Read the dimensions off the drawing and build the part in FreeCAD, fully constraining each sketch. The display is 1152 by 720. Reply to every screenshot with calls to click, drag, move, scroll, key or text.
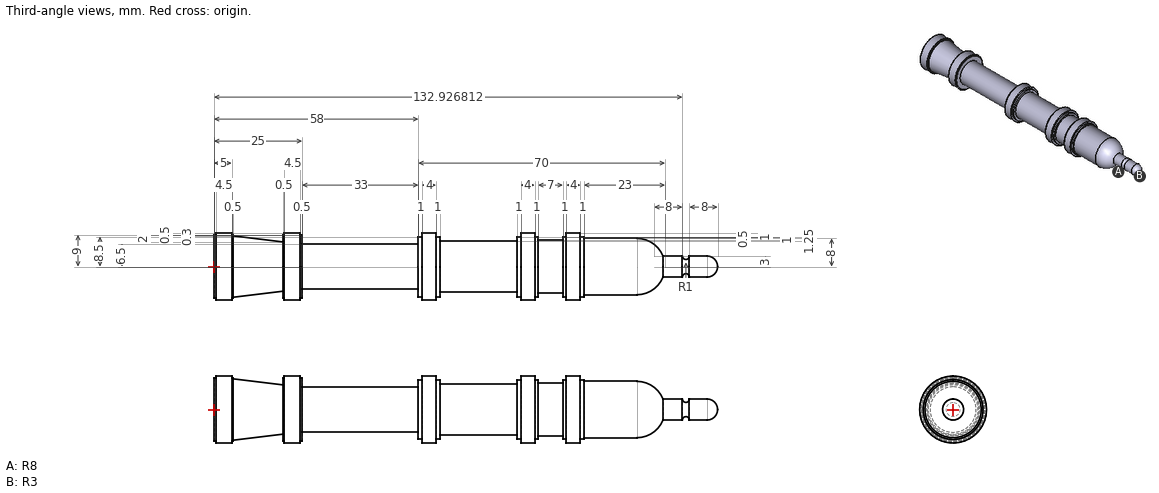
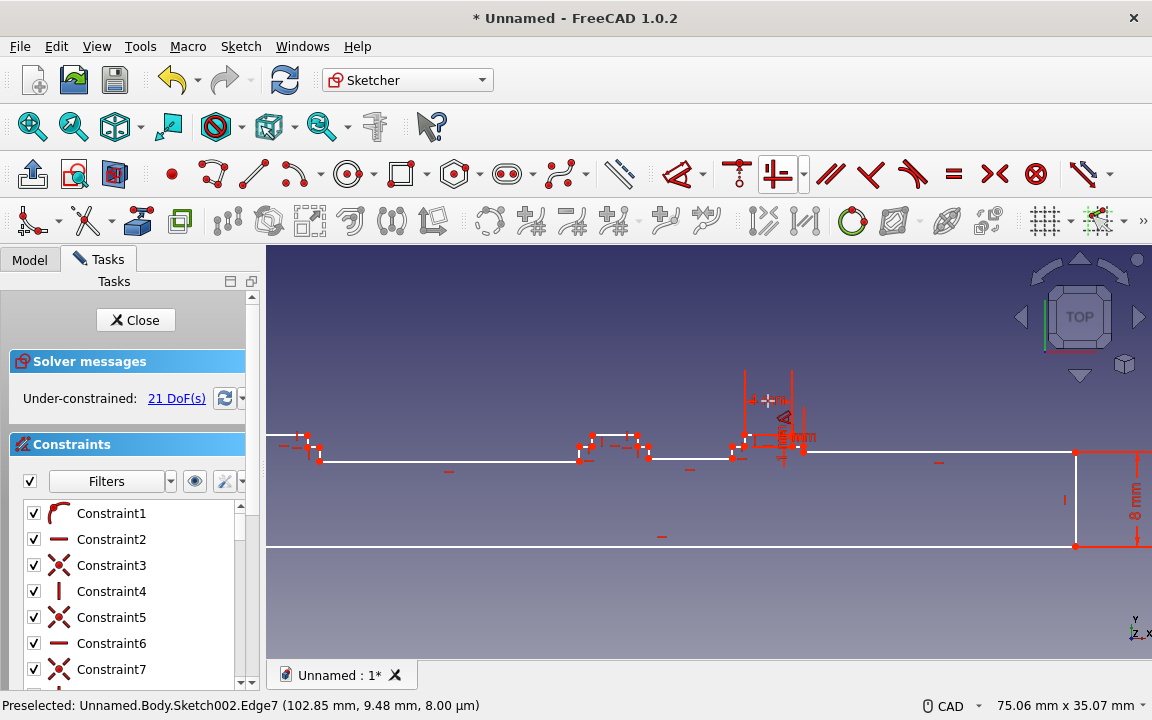
scroll(745, 441, up, 7)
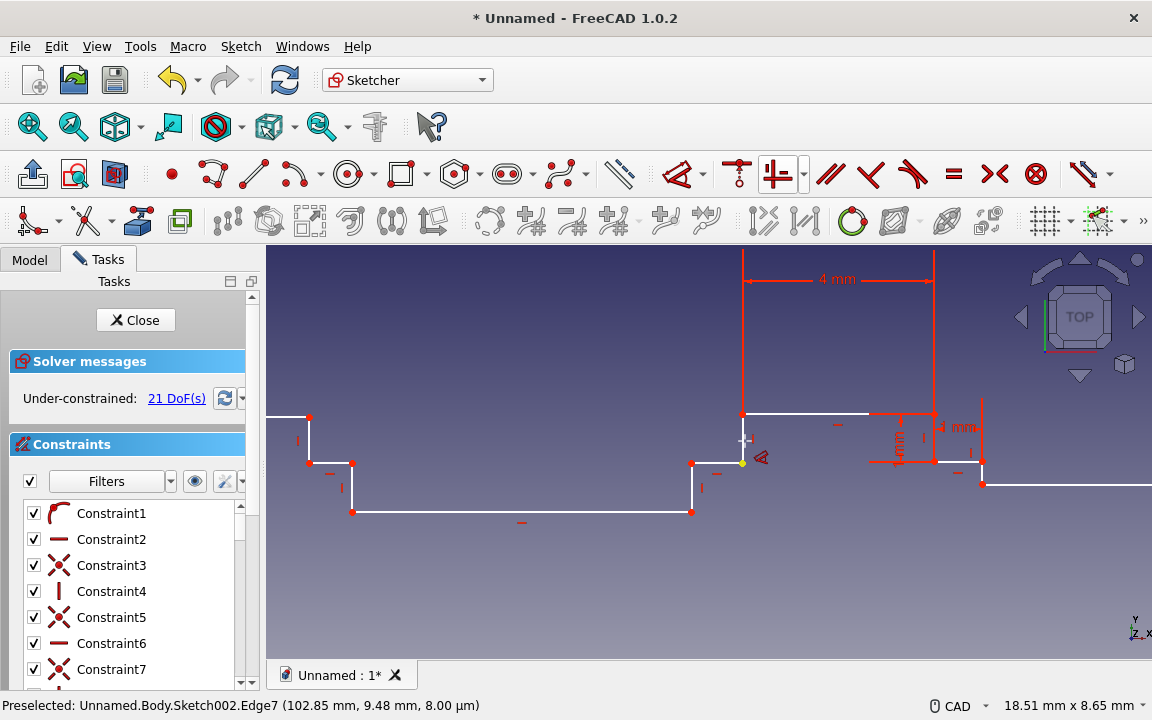
click(743, 439)
click(777, 439)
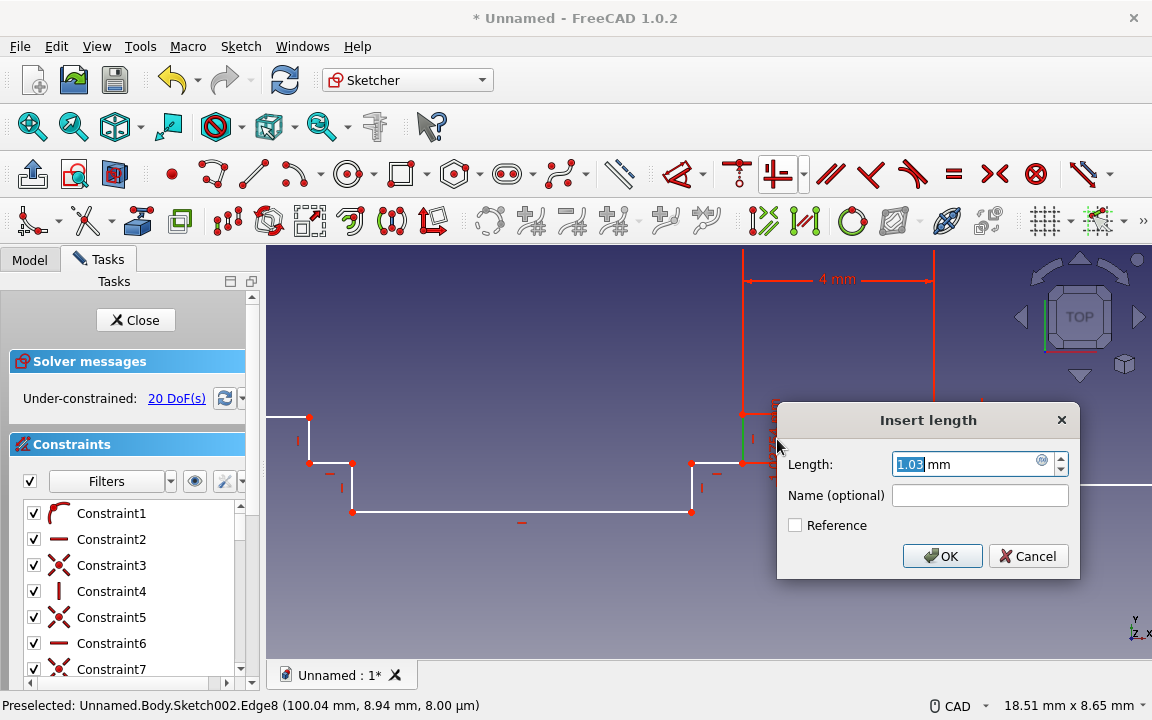
text(1)
key(Return)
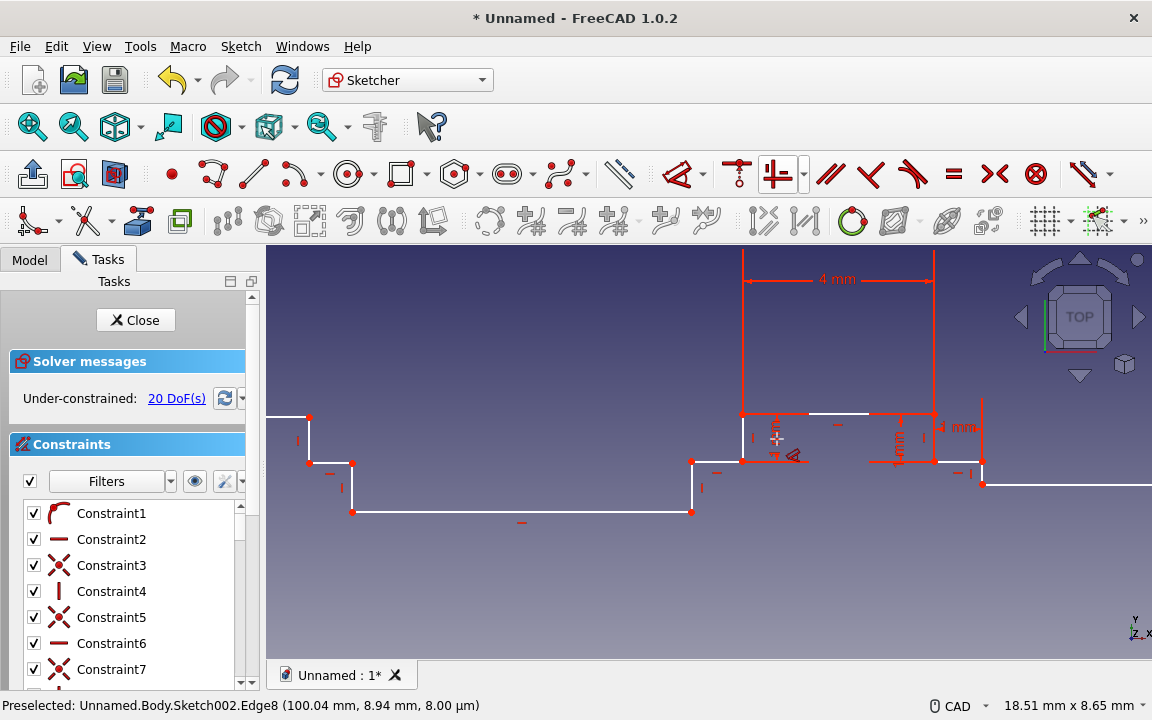
click(728, 462)
click(706, 428)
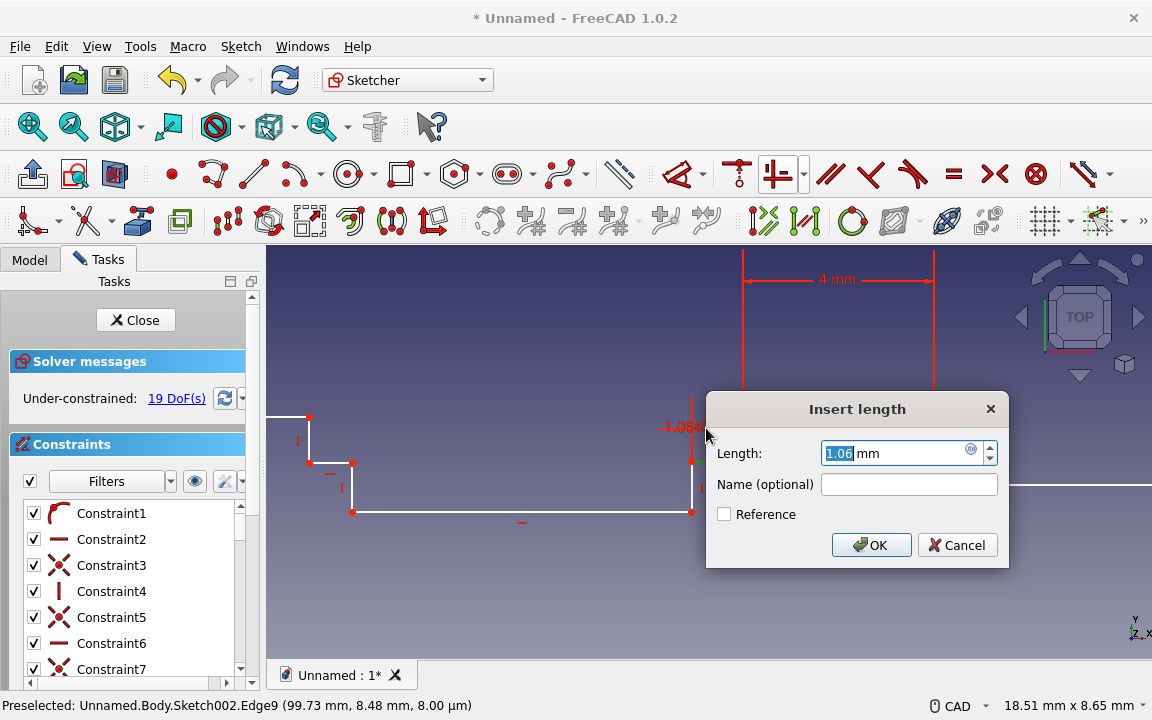
text(1)
key(Return)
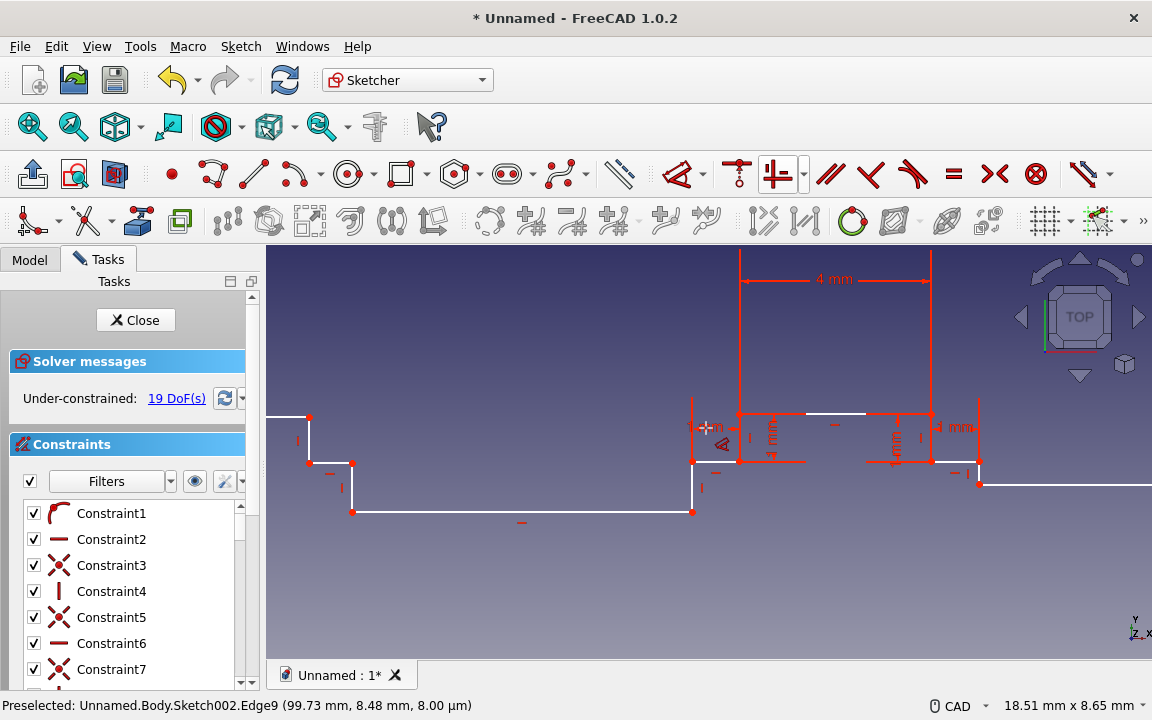
click(692, 477)
click(726, 487)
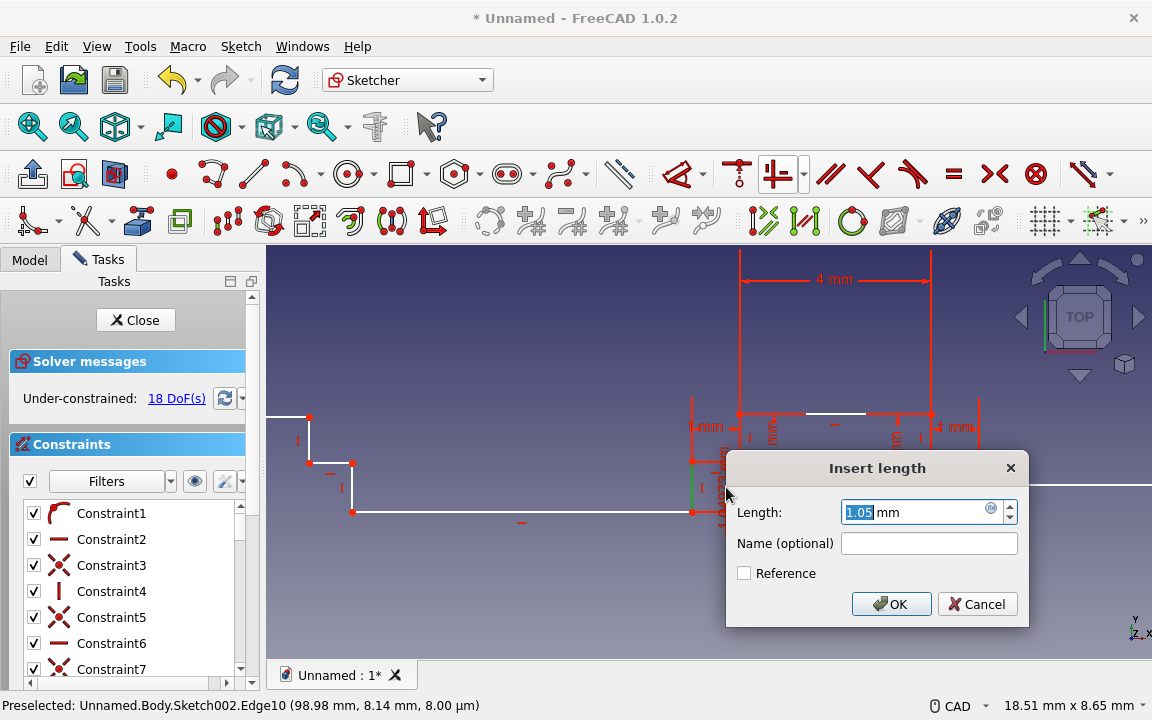
text(1)
key(Return)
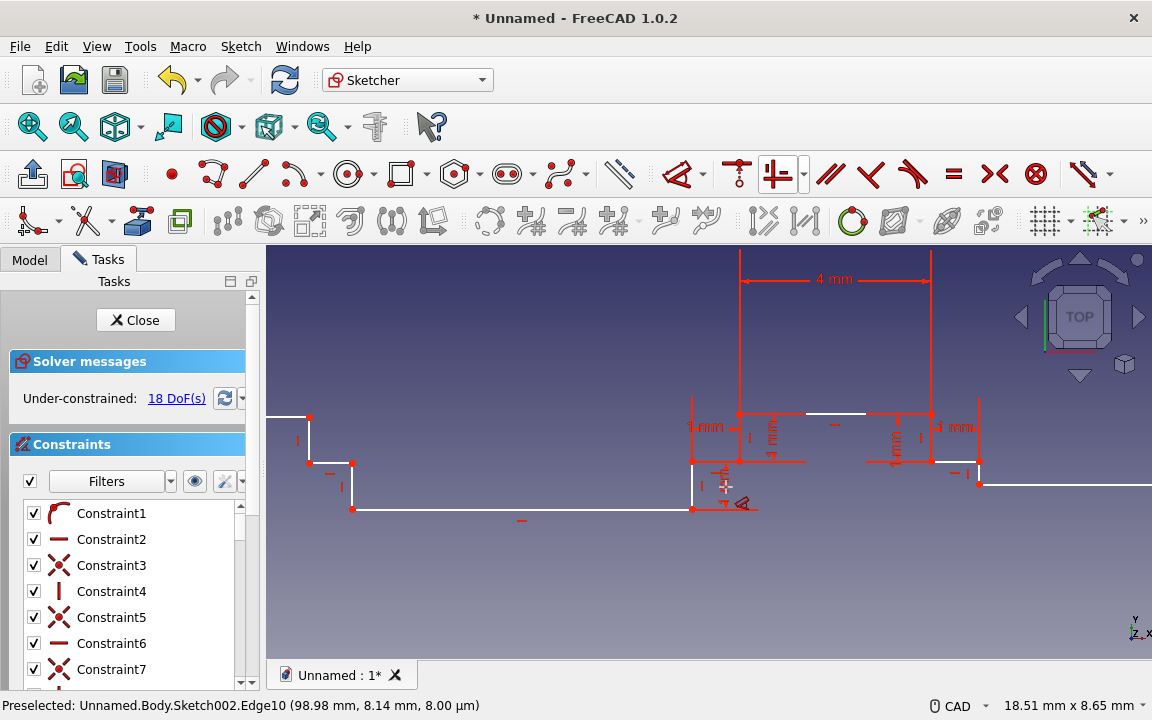
scroll(771, 437, down, 13)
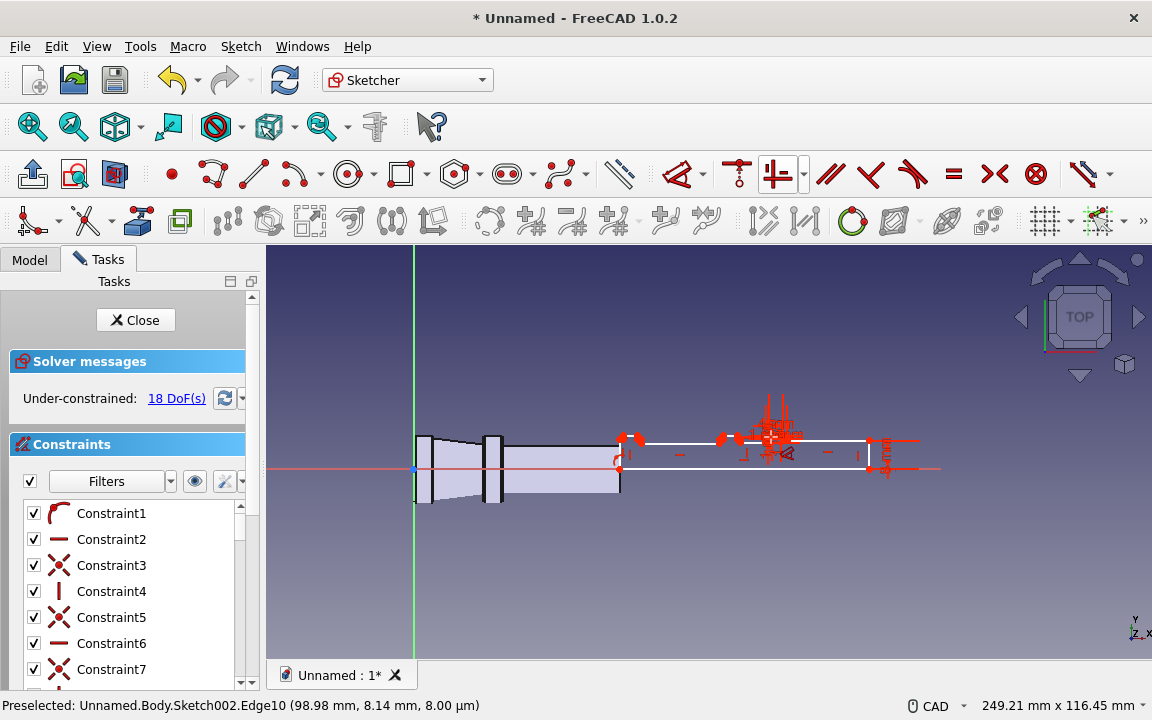
scroll(758, 443, up, 4)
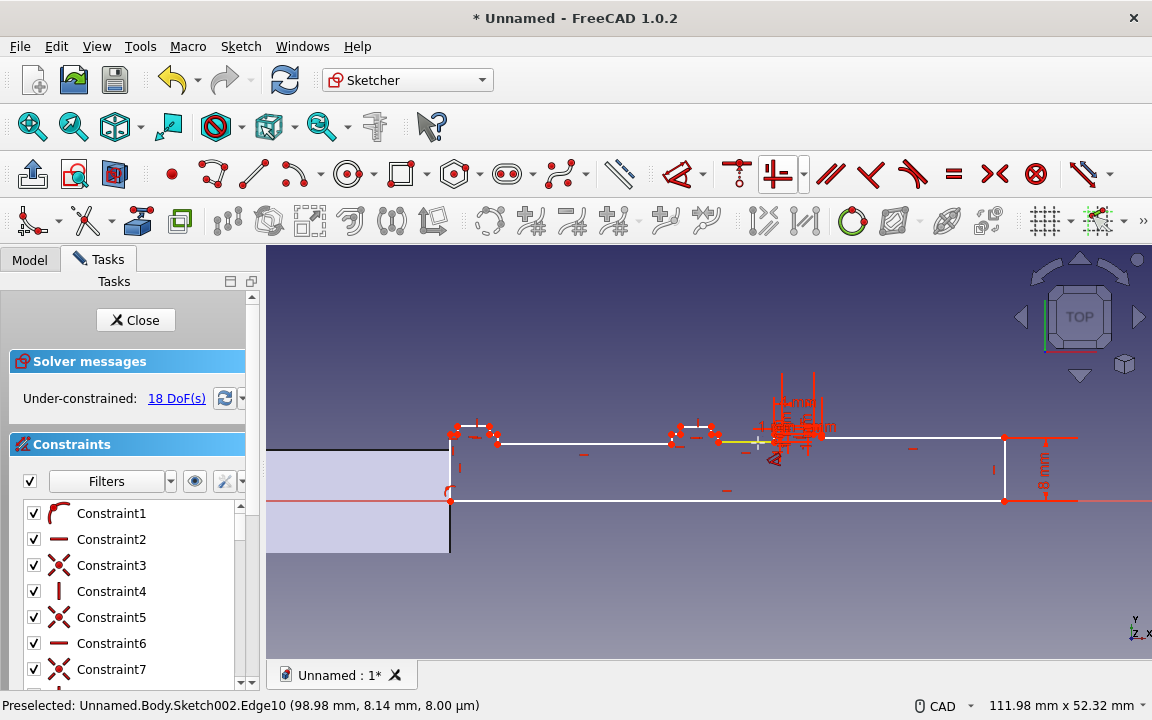
click(758, 442)
click(727, 408)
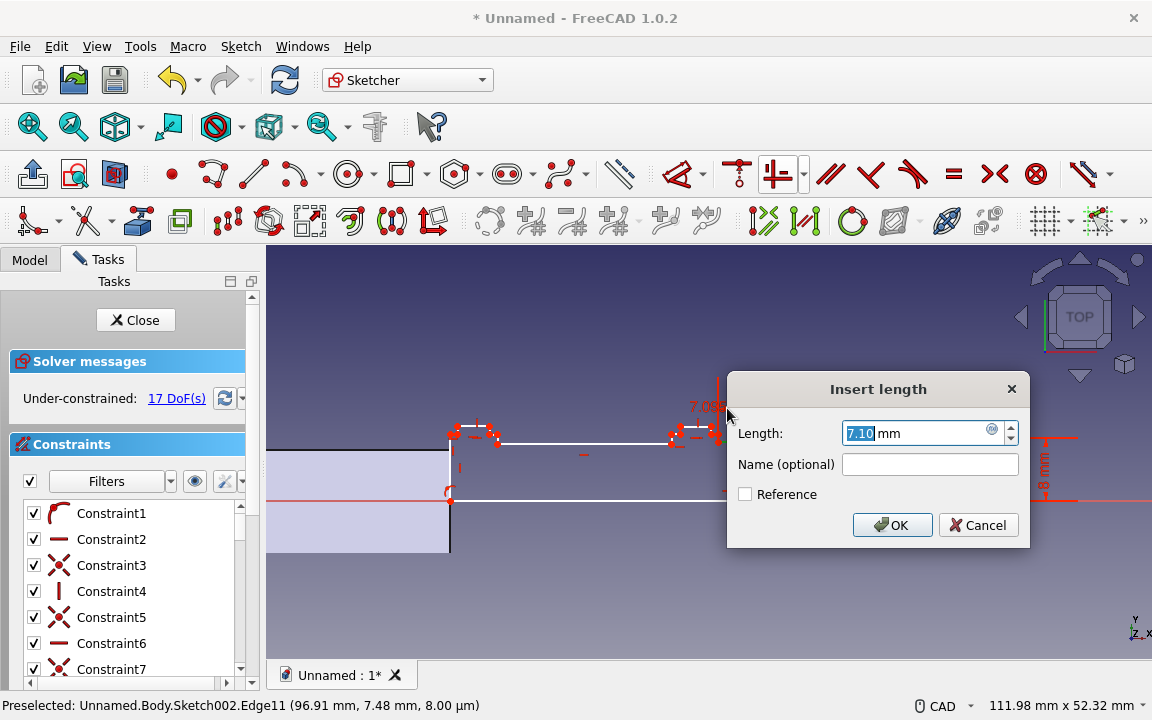
text(7)
key(Return)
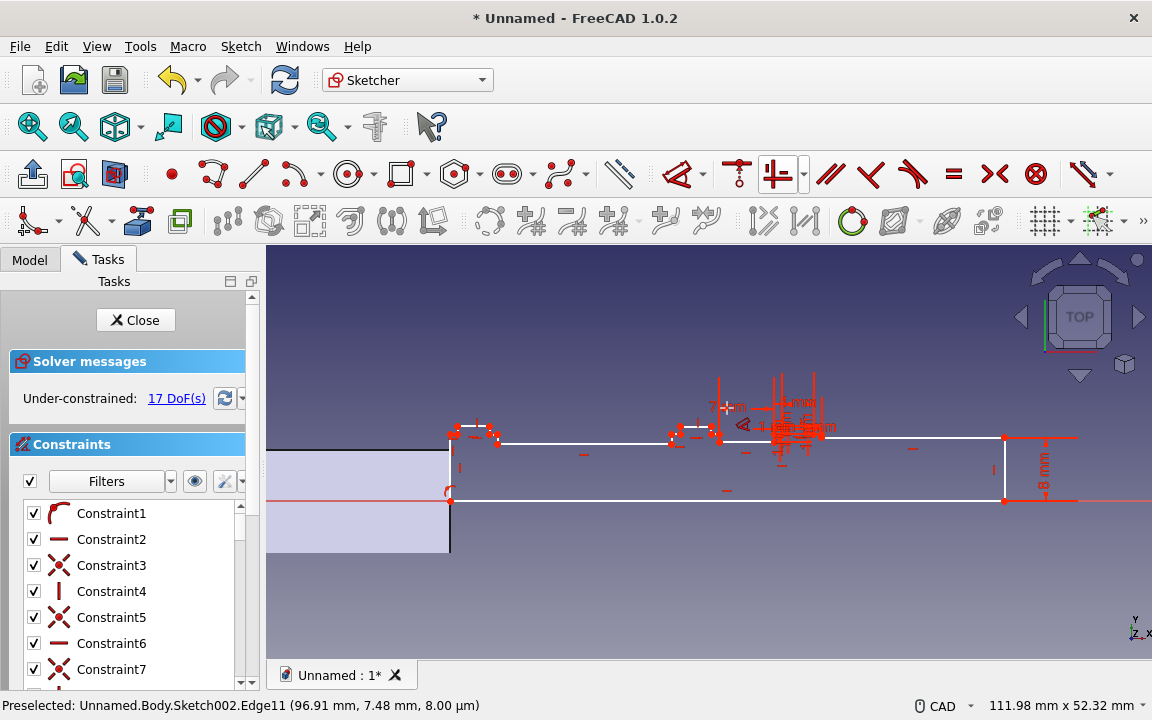
scroll(719, 438, up, 9)